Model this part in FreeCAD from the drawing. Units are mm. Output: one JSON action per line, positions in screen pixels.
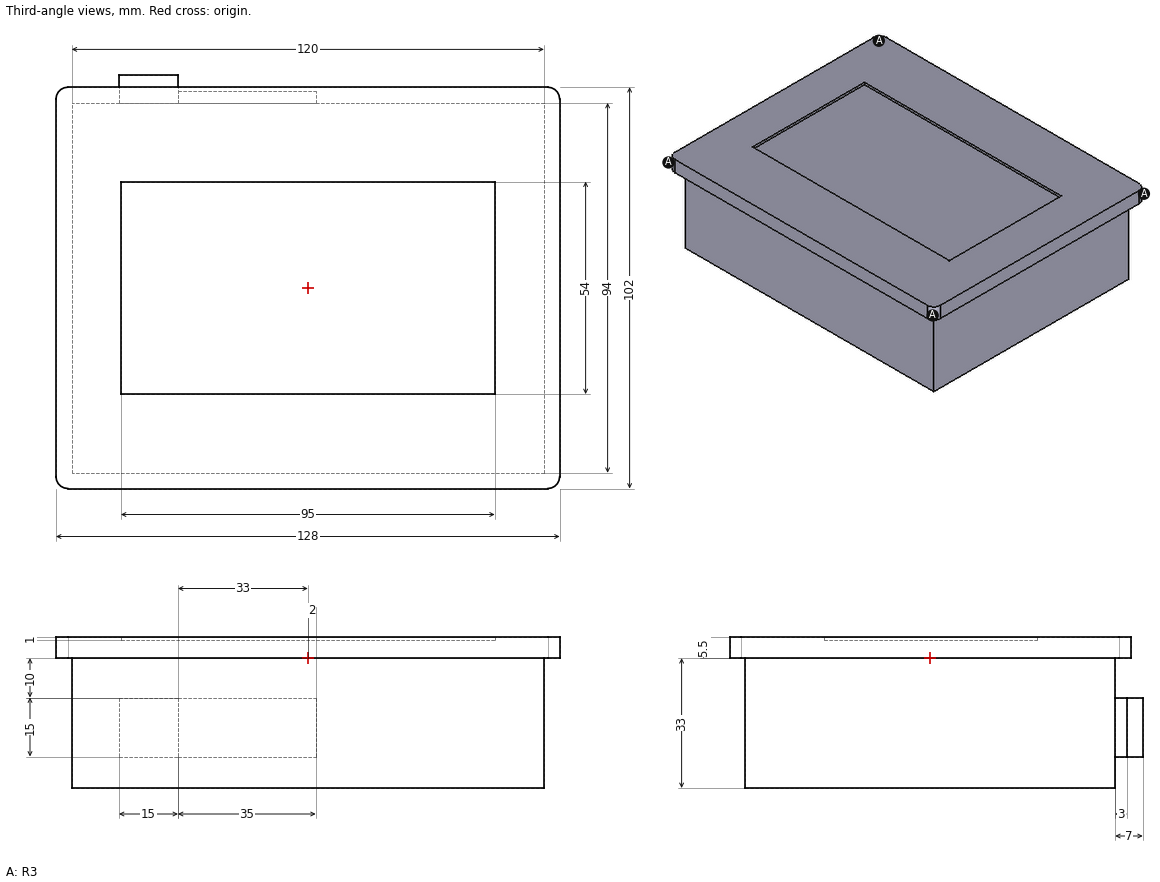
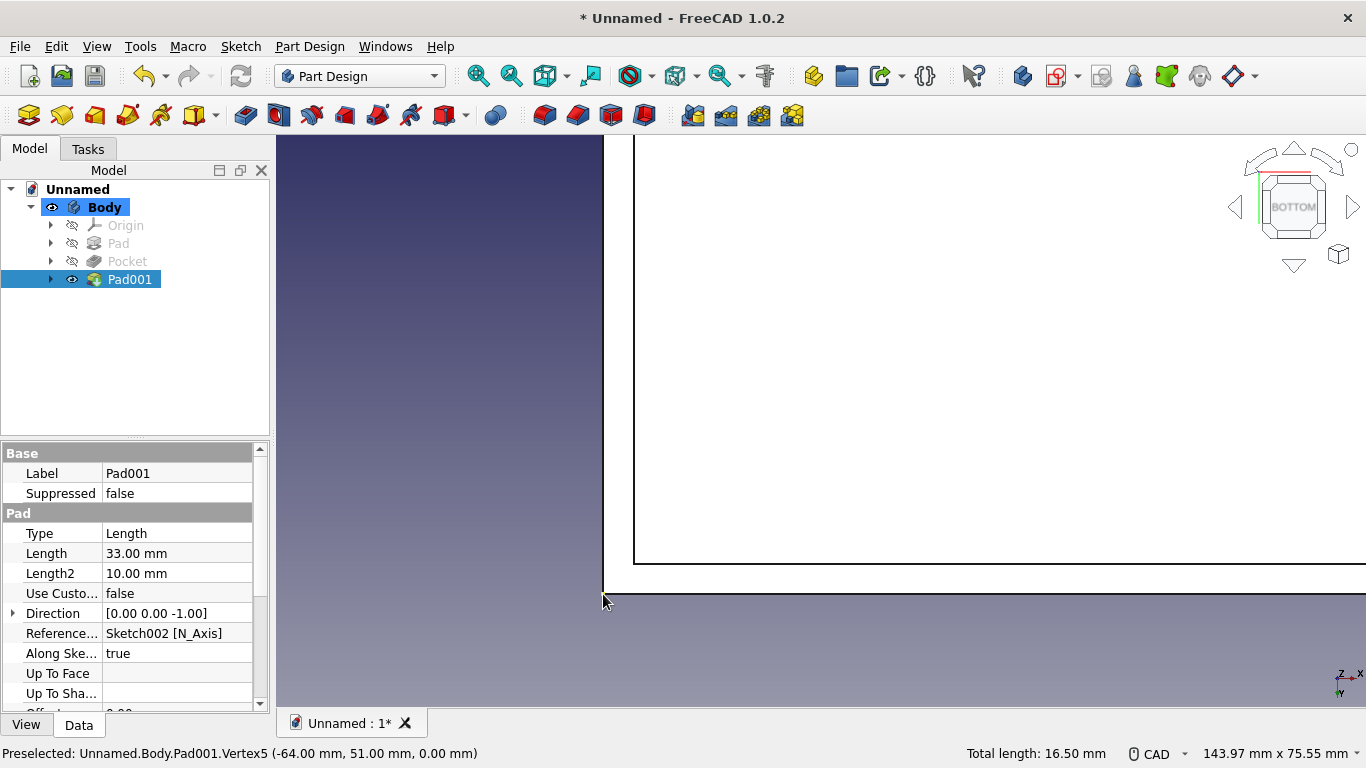
{"action": "key", "text": "v f"}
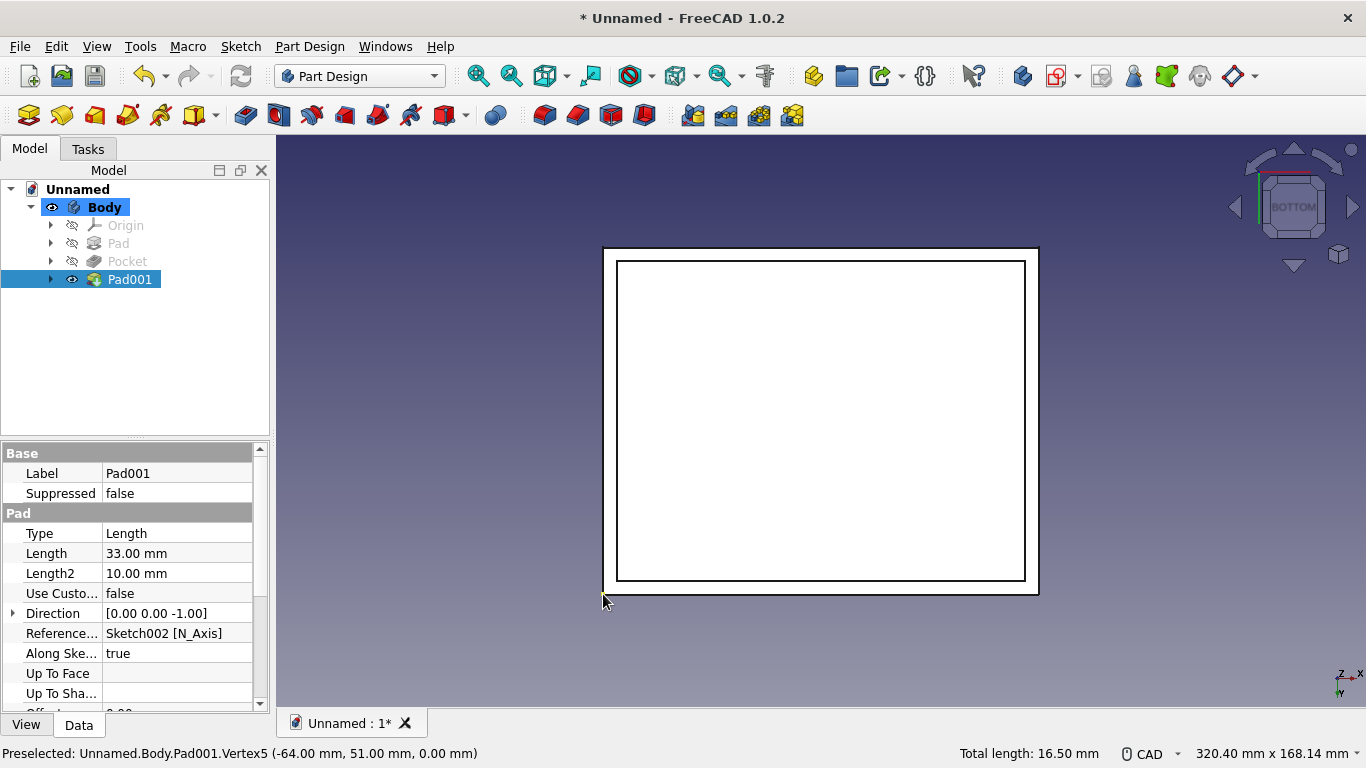
{"action": "key", "text": "4"}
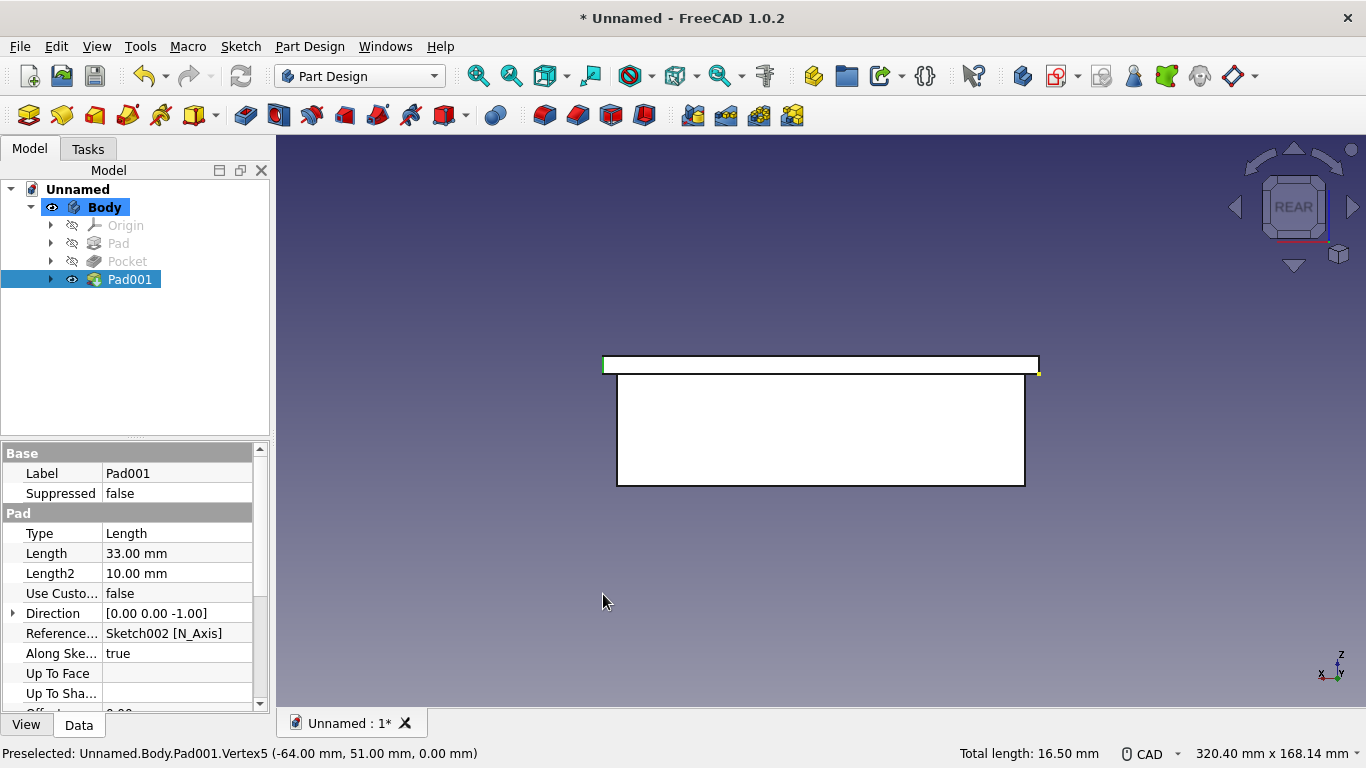
{"action": "left_click", "coordinate": [479, 76]}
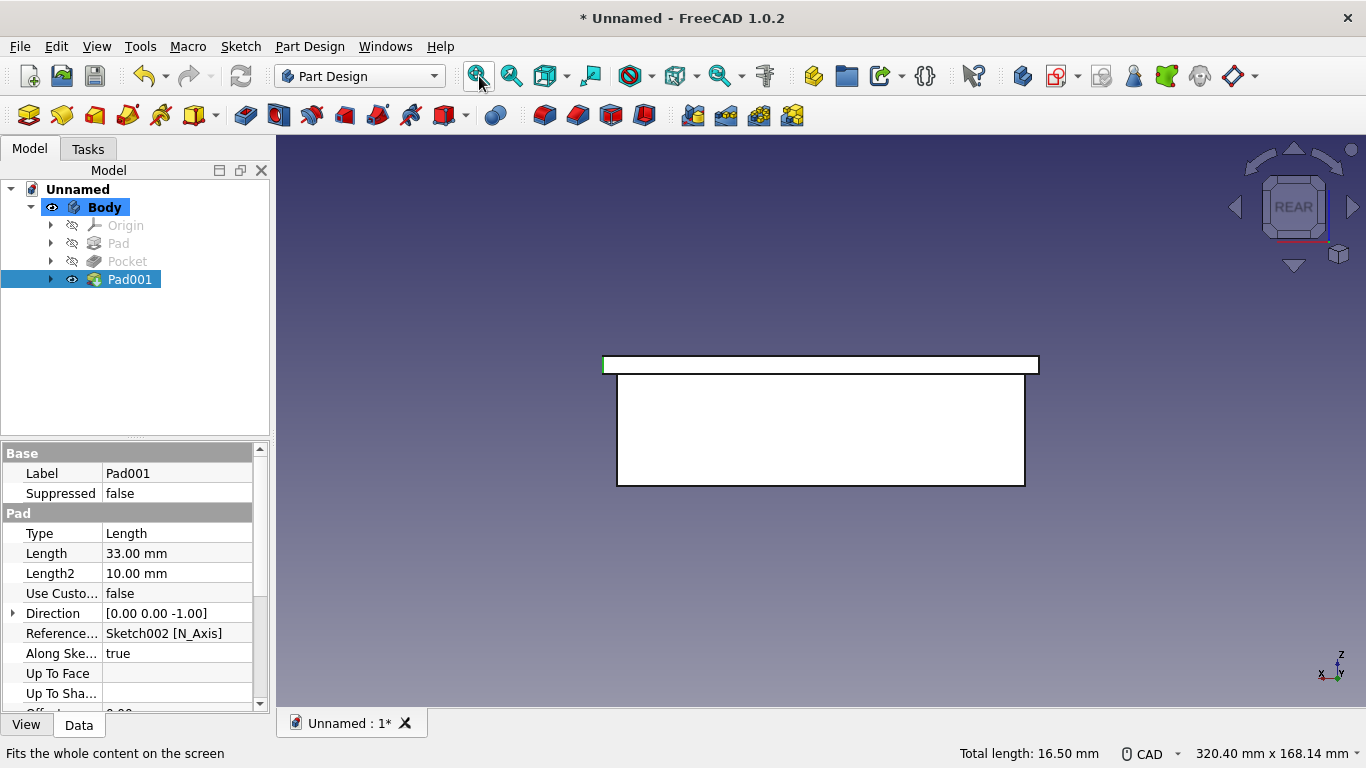
{"action": "left_click", "coordinate": [1039, 364], "text": "ctrl"}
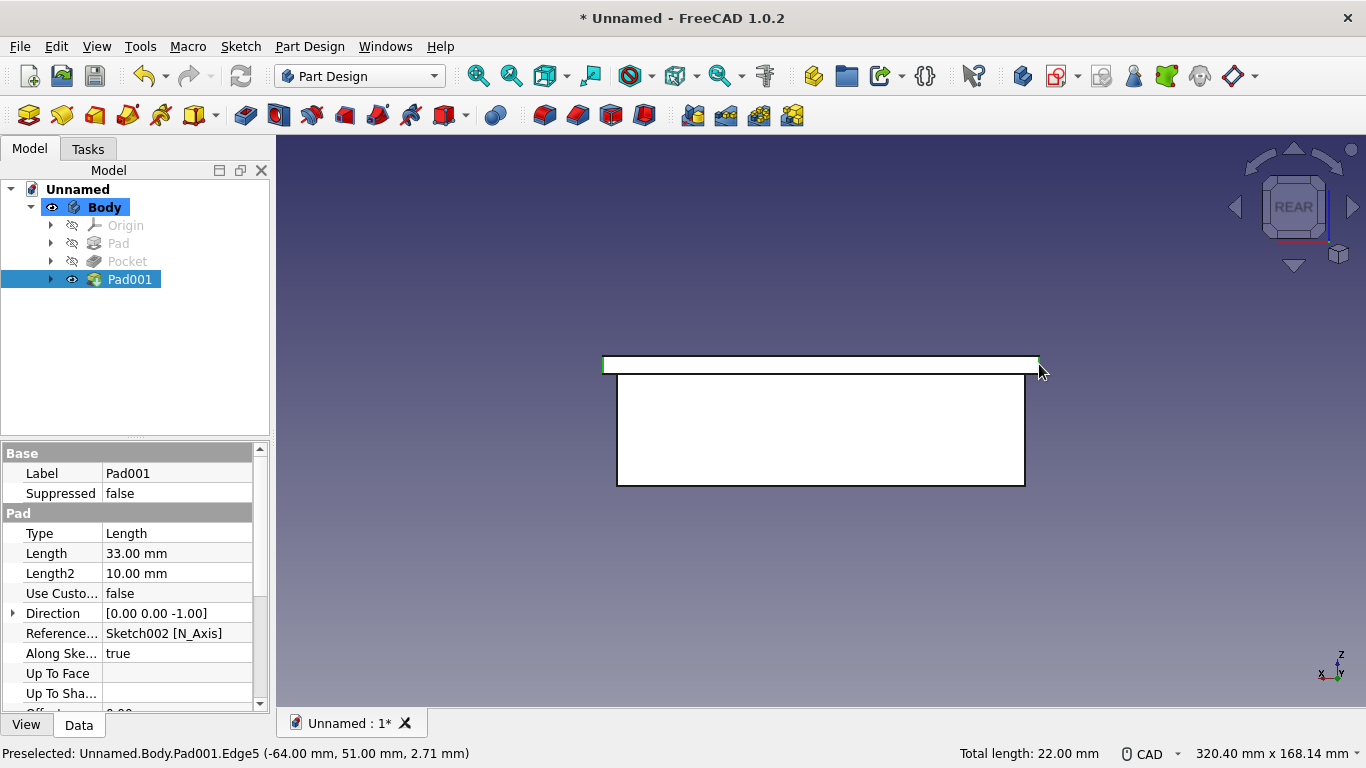
{"action": "left_click", "coordinate": [545, 116]}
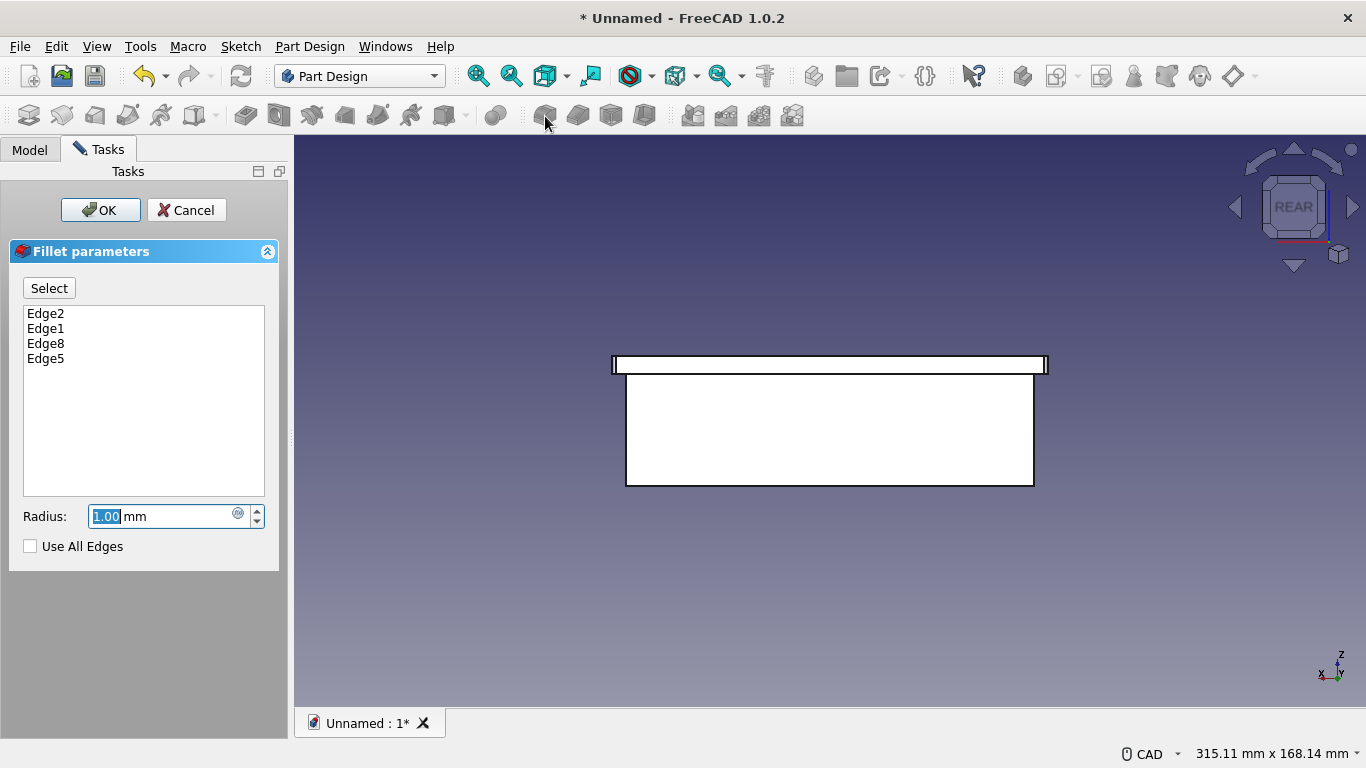
{"action": "type", "text": "3"}
{"action": "key", "text": "Tab"}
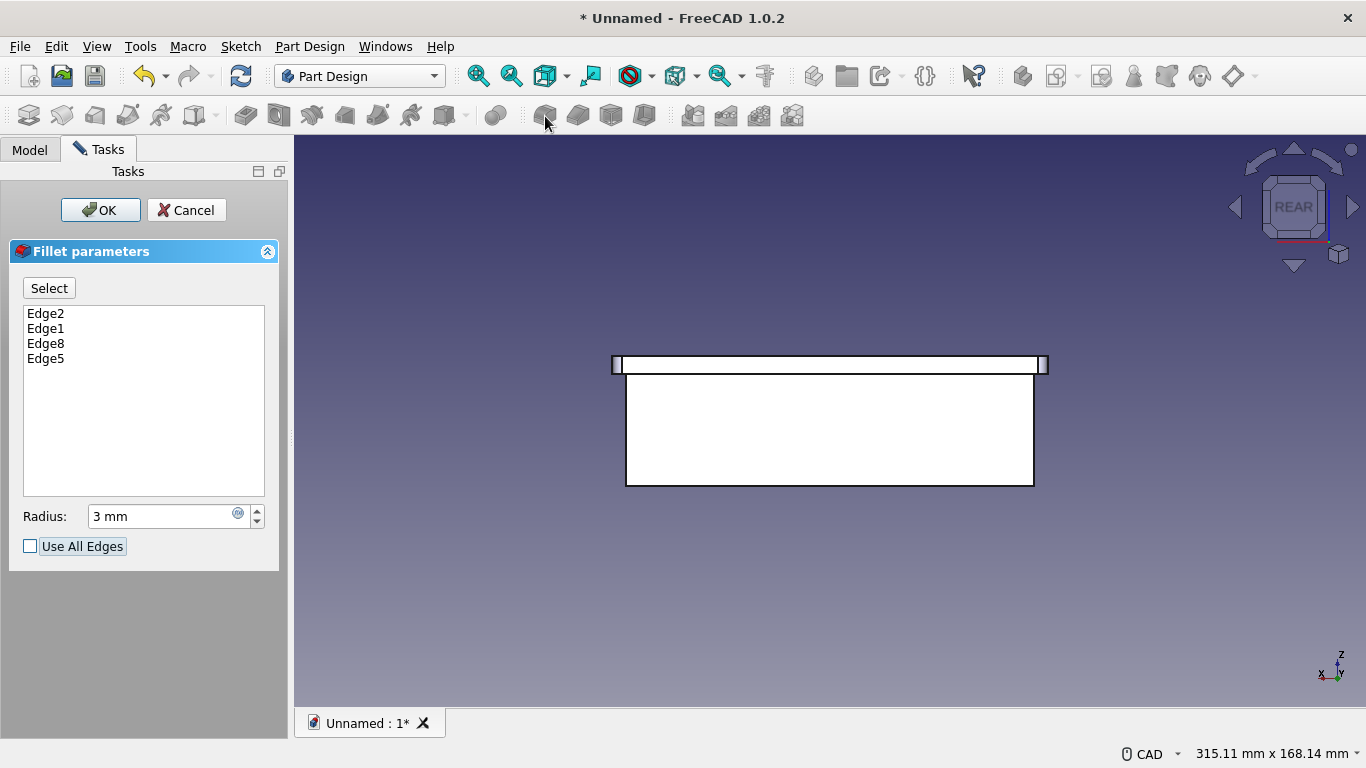
{"action": "left_click", "coordinate": [101, 210]}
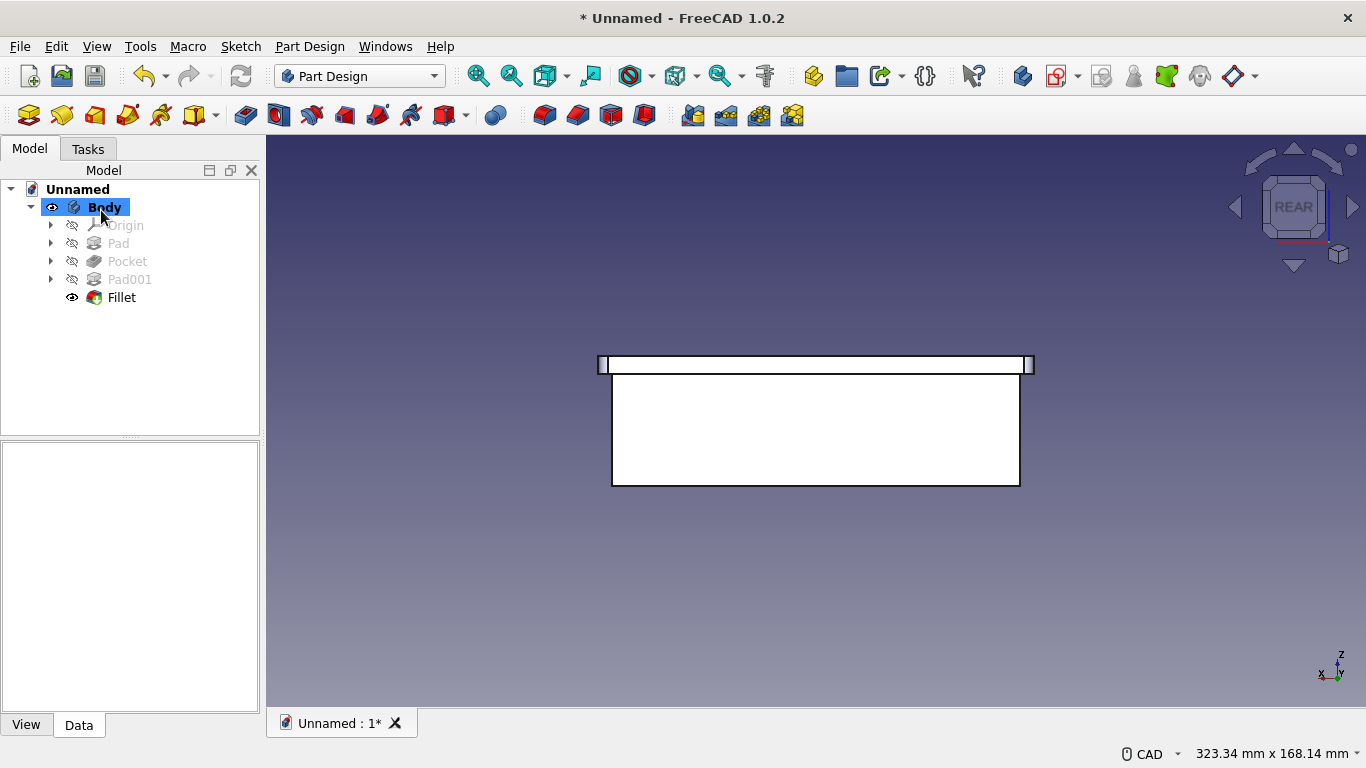
{"action": "key", "text": "v f"}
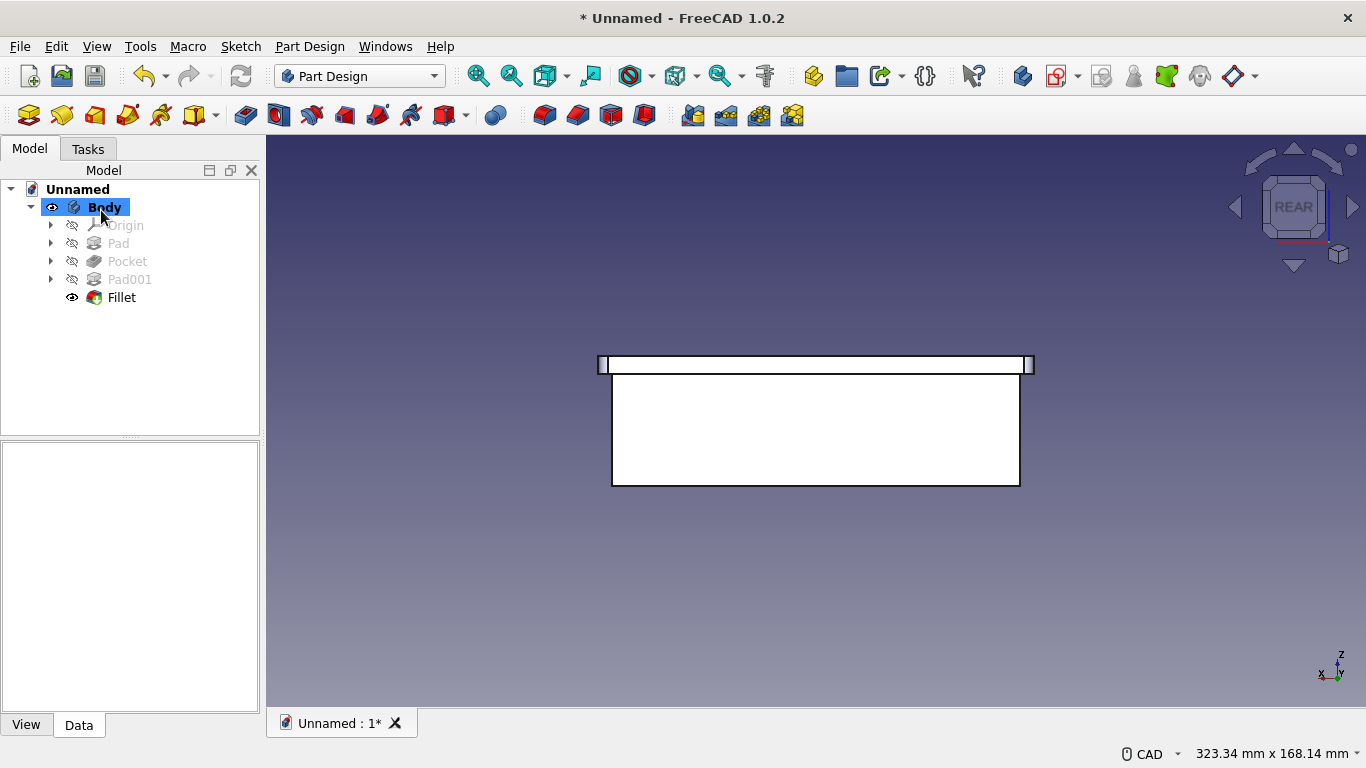
{"action": "left_click", "coordinate": [699, 429]}